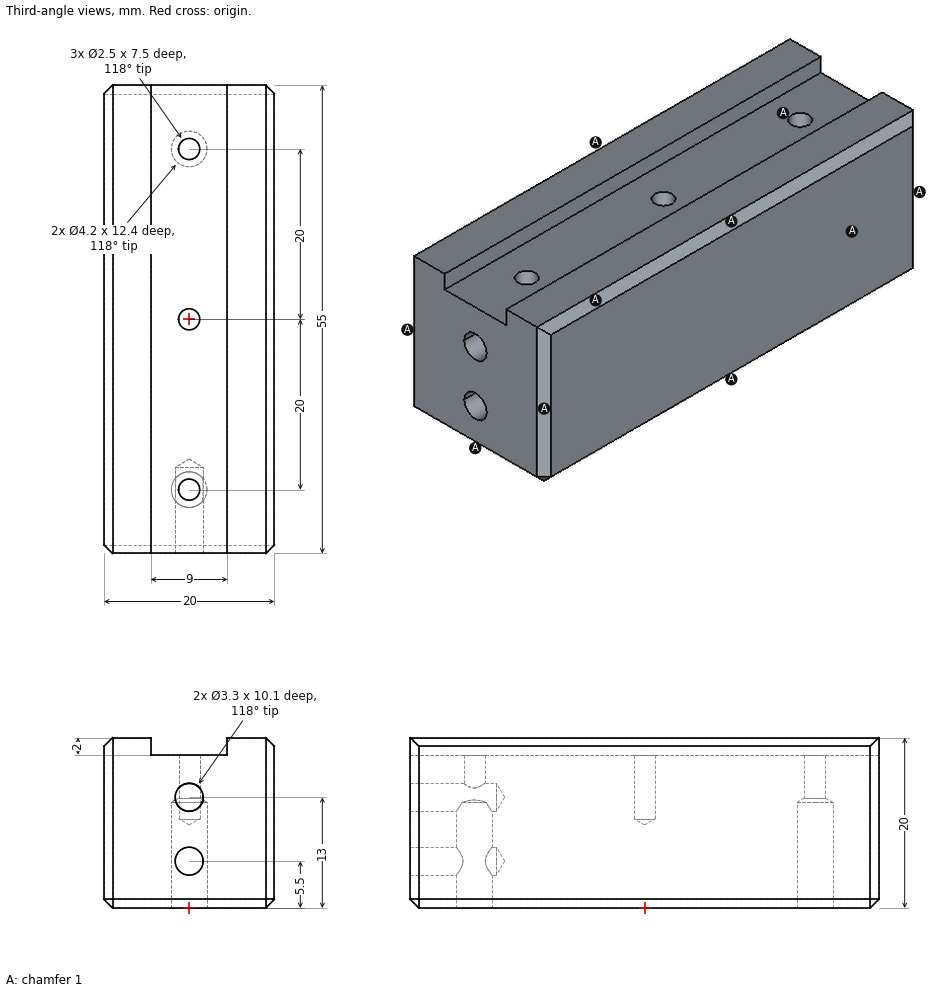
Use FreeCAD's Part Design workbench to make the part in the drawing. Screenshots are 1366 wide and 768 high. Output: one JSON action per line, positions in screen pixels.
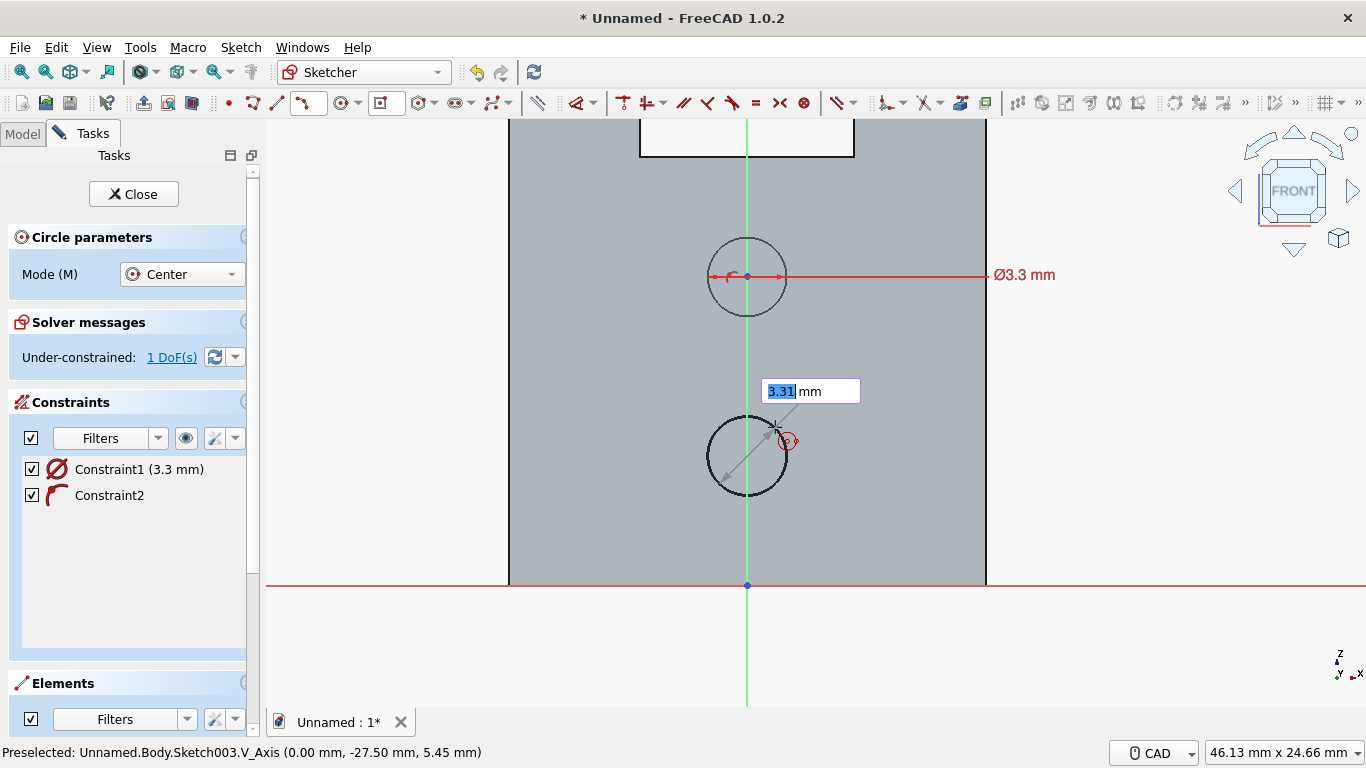
{"action": "type", "text": "3.3"}
{"action": "key", "text": "Return"}
{"action": "key", "text": "Escape"}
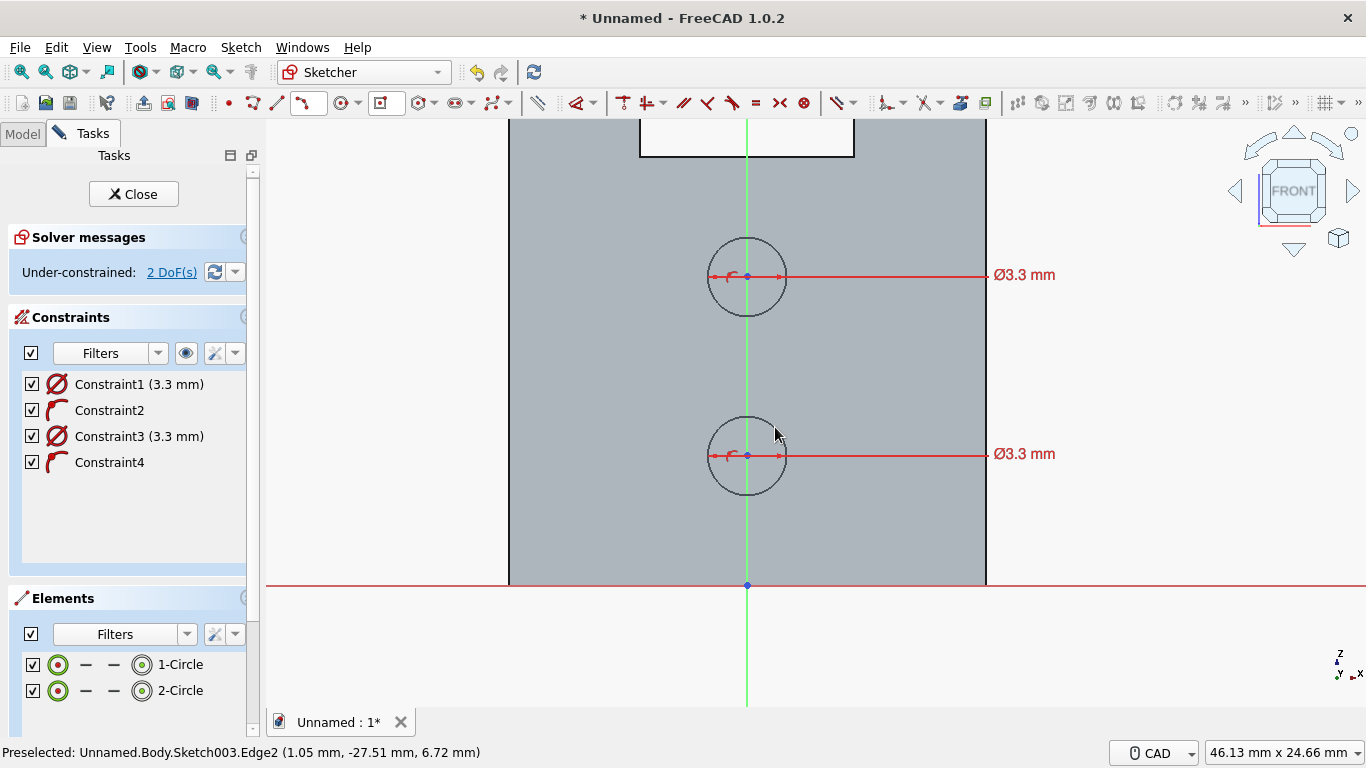
{"action": "left_click", "coordinate": [576, 104]}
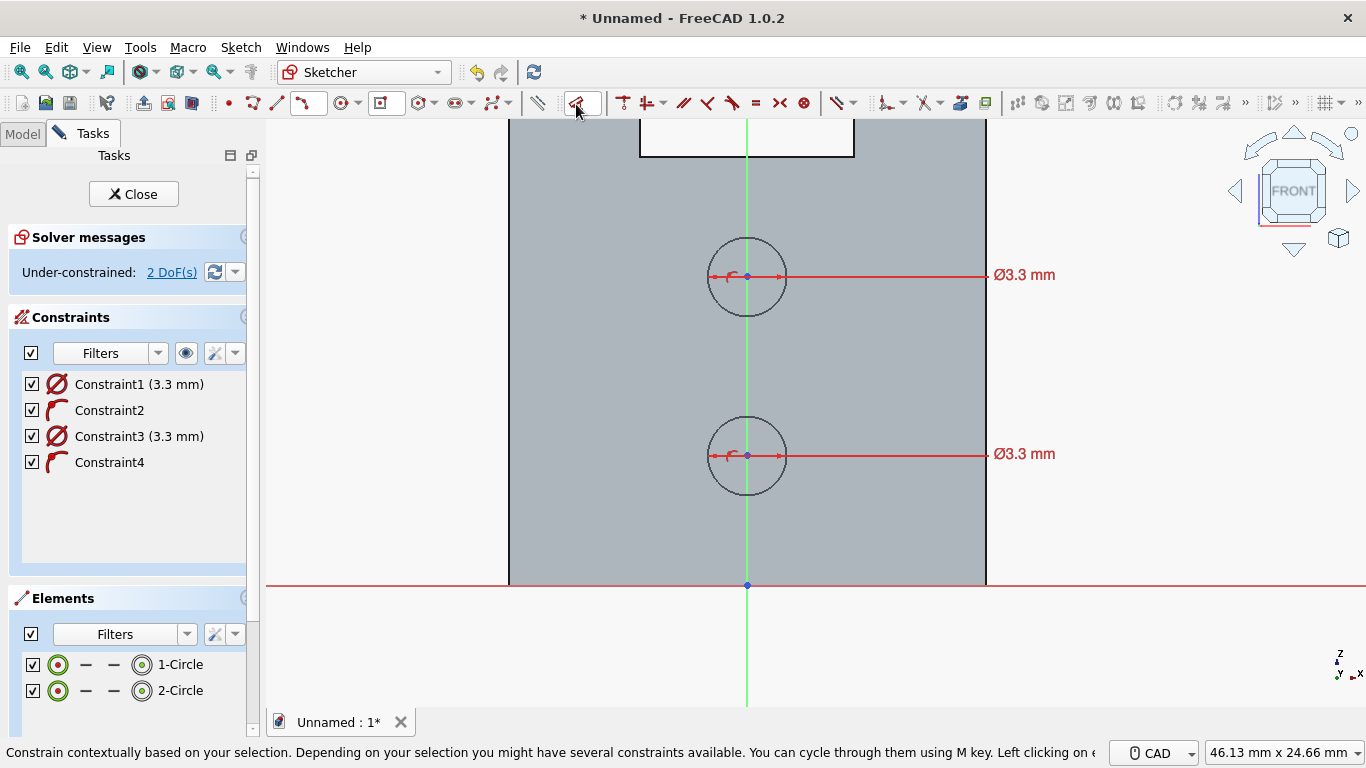
{"action": "left_click", "coordinate": [747, 277]}
{"action": "left_click", "coordinate": [781, 360]}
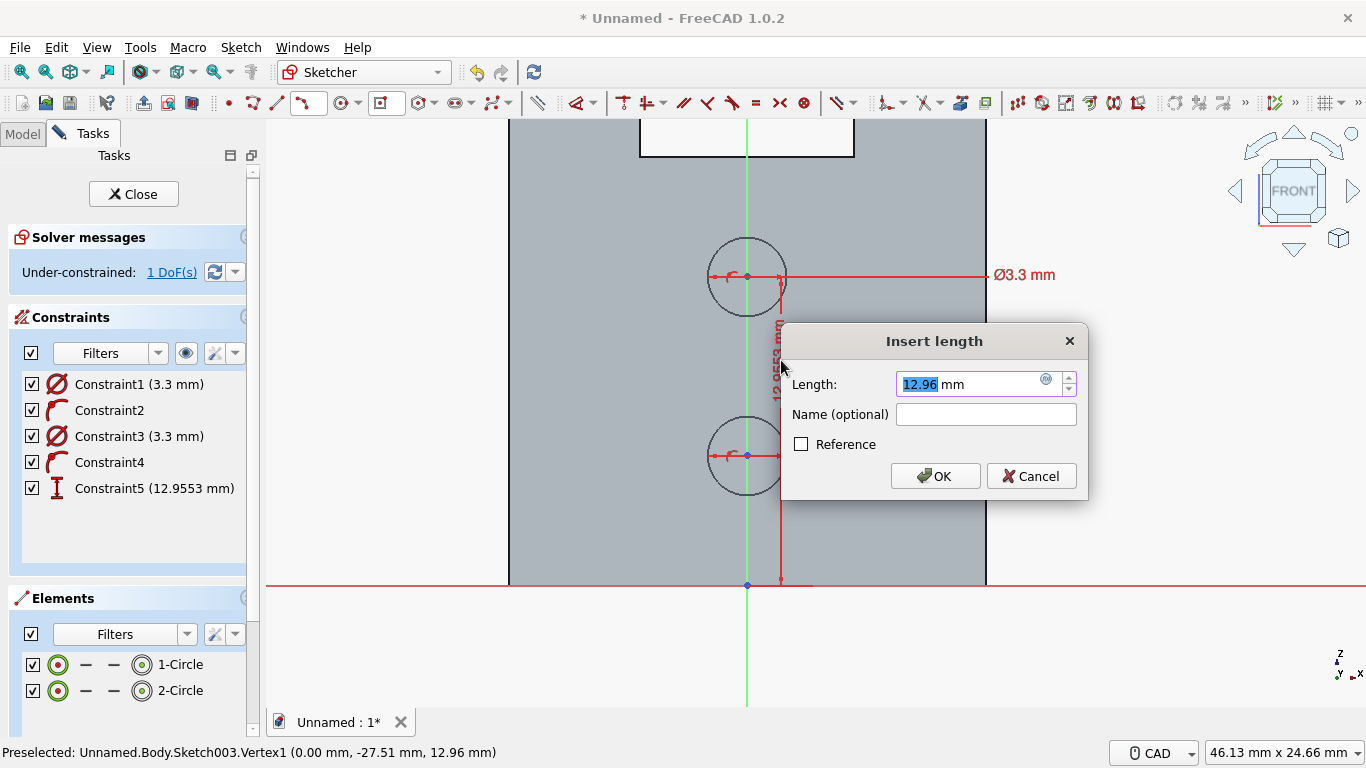
{"action": "type", "text": "13"}
{"action": "key", "text": "Return"}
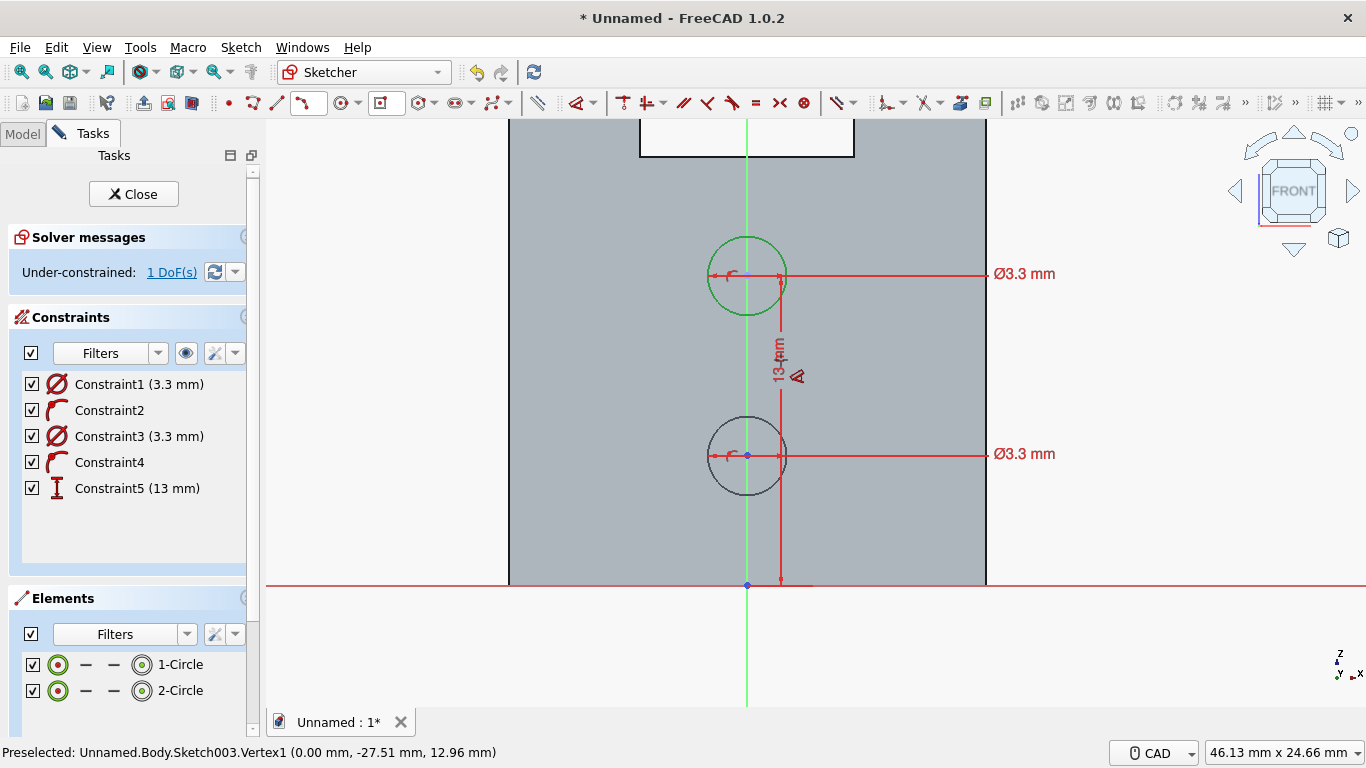
{"action": "left_click", "coordinate": [747, 456]}
{"action": "left_click", "coordinate": [781, 521]}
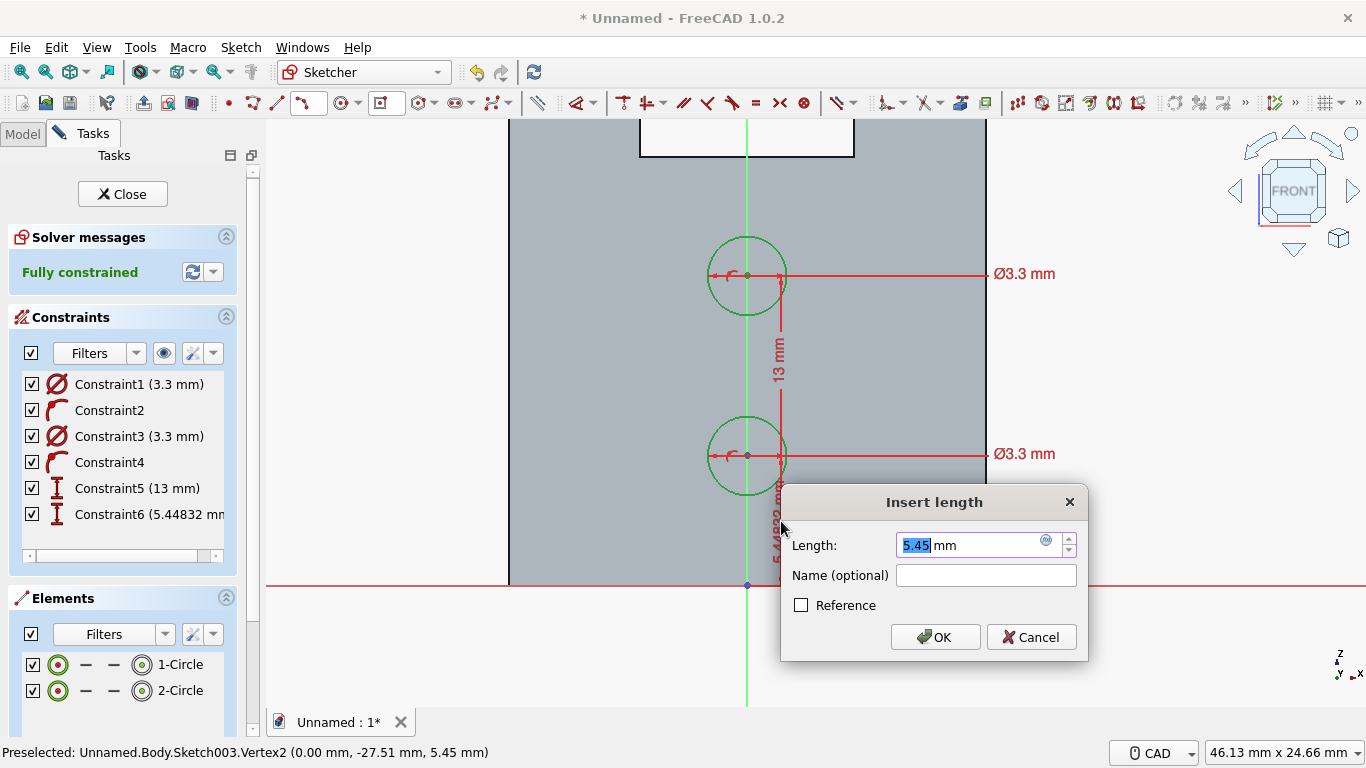
{"action": "type", "text": "5.5"}
{"action": "key", "text": "Return"}
{"action": "key", "text": "Escape"}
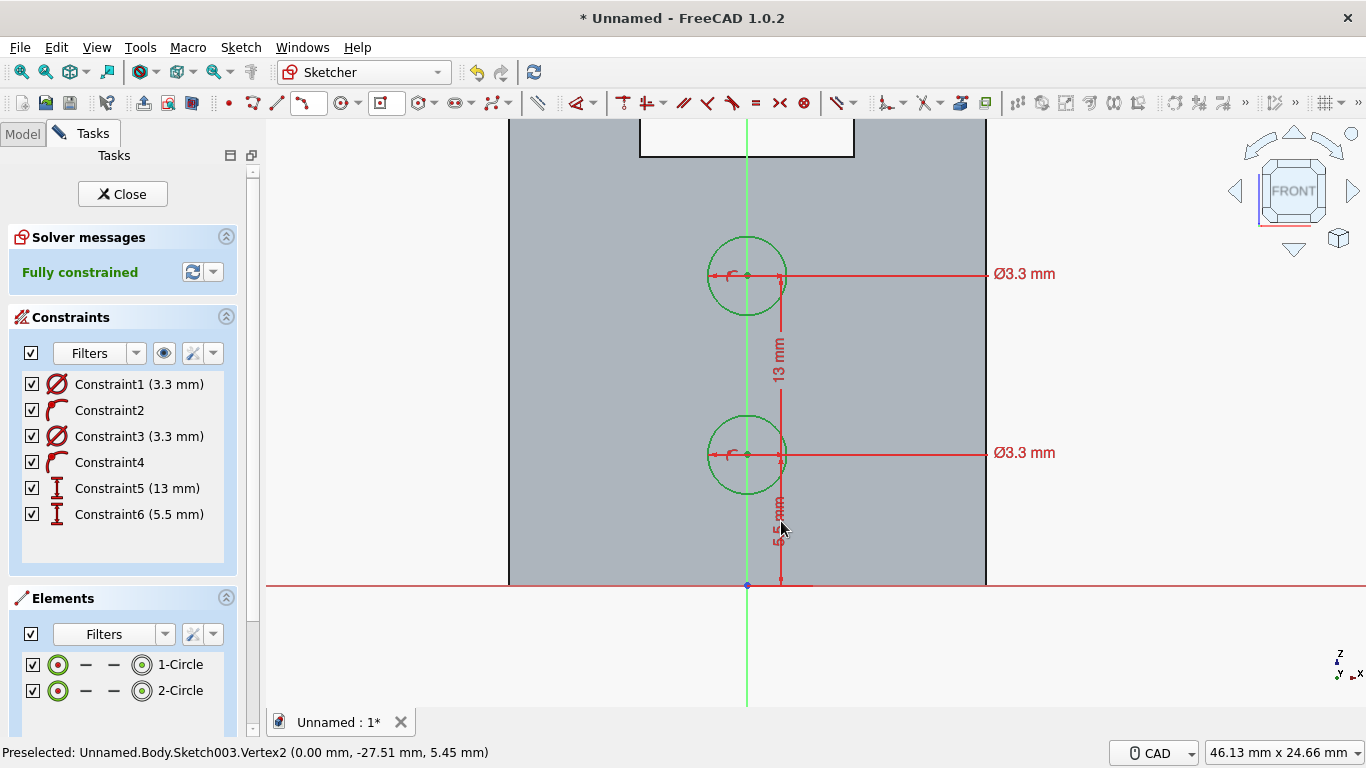
{"action": "left_click", "coordinate": [123, 194]}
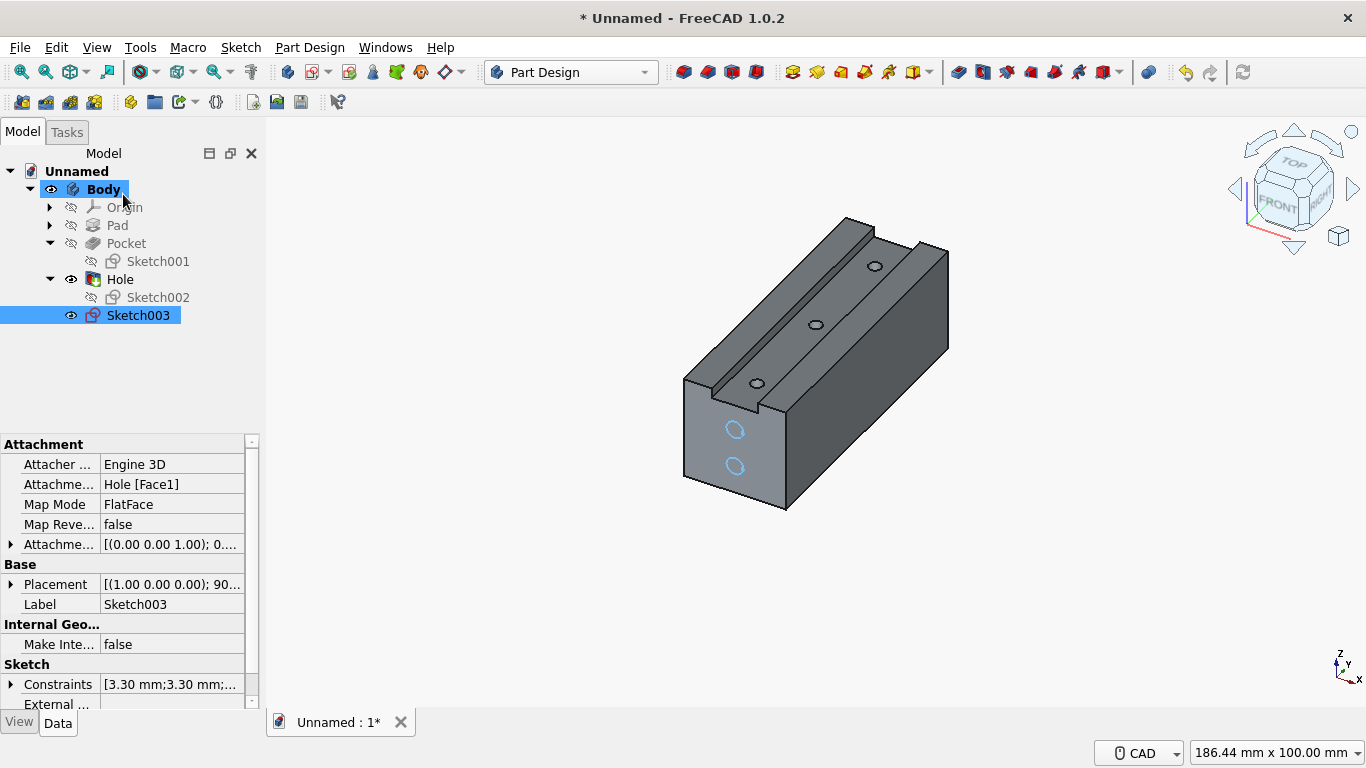
{"action": "left_click", "coordinate": [984, 72]}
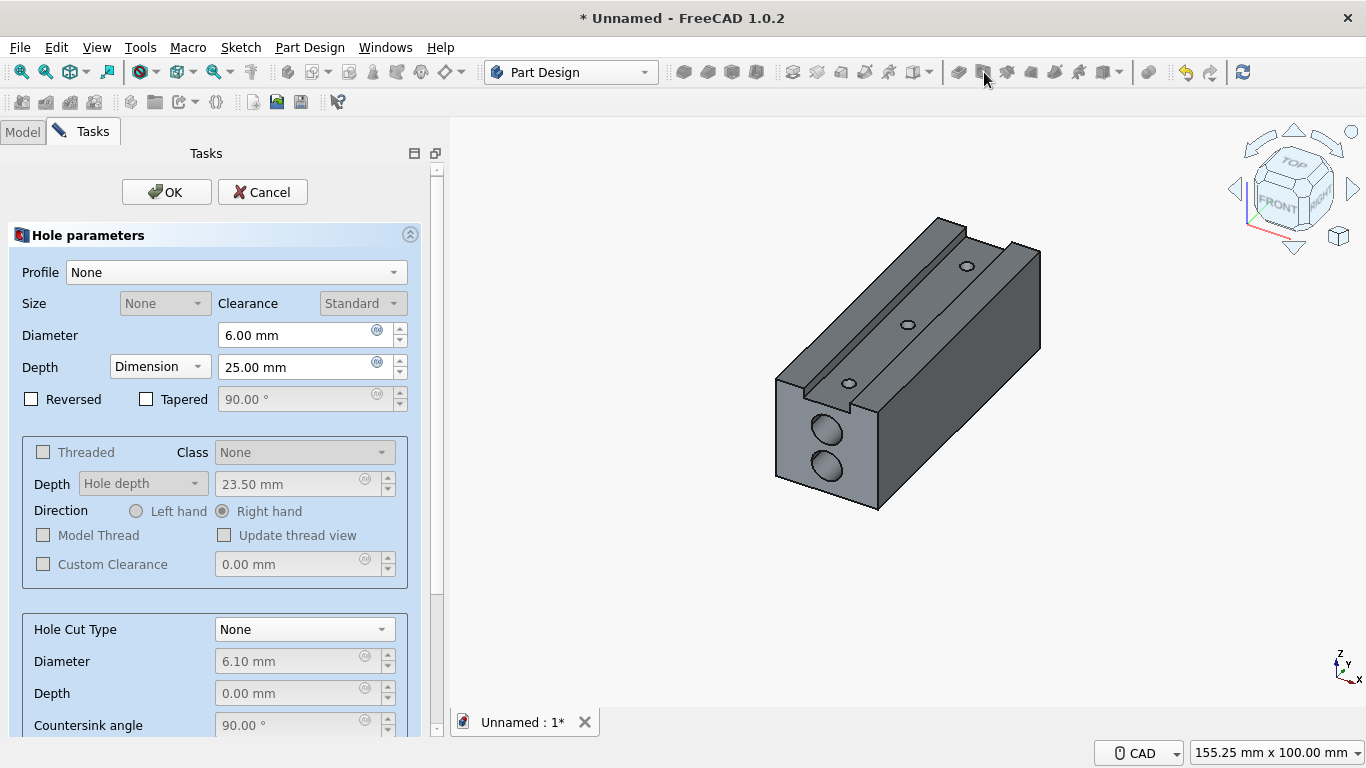
{"action": "triple_click", "coordinate": [305, 335]}